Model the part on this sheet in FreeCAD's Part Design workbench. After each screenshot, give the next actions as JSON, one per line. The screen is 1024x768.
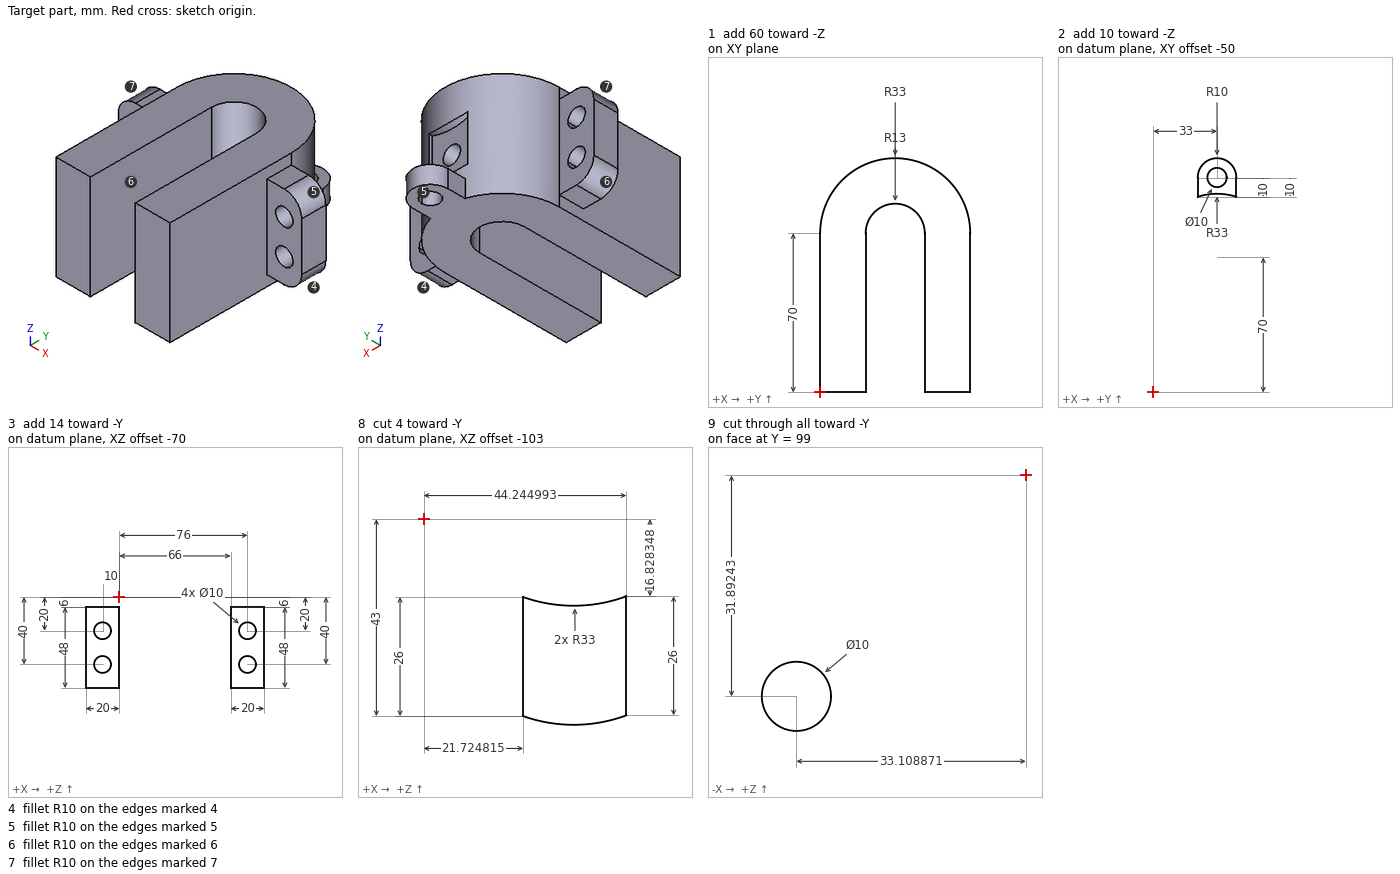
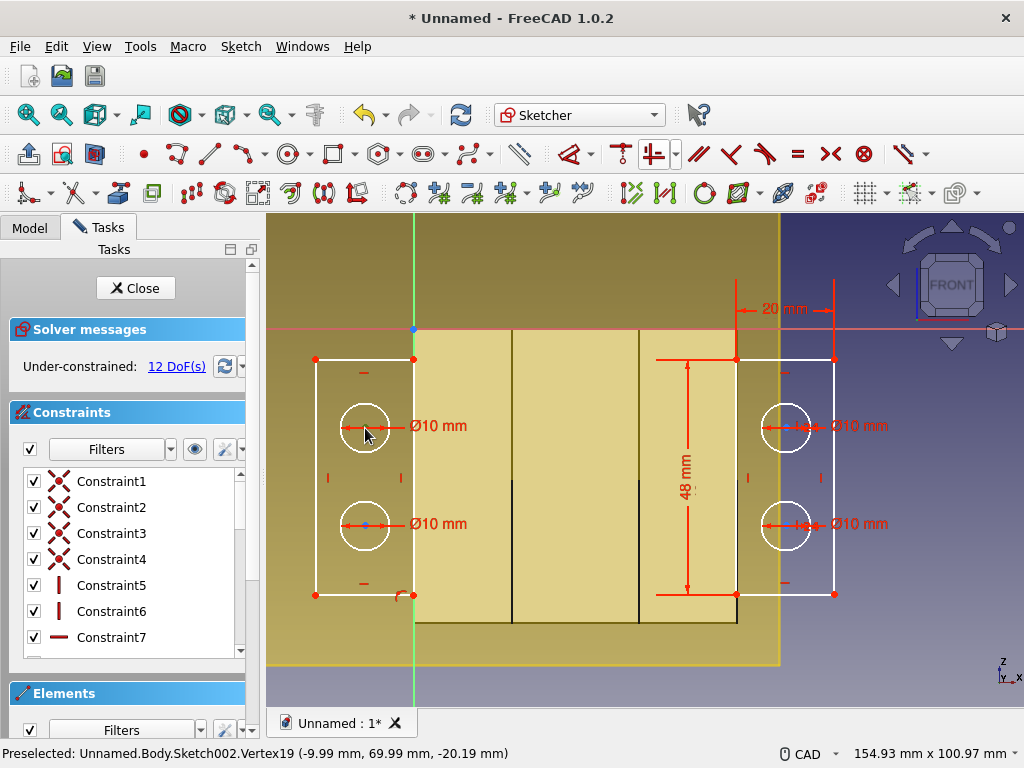
{"action": "left_click", "coordinate": [365, 526]}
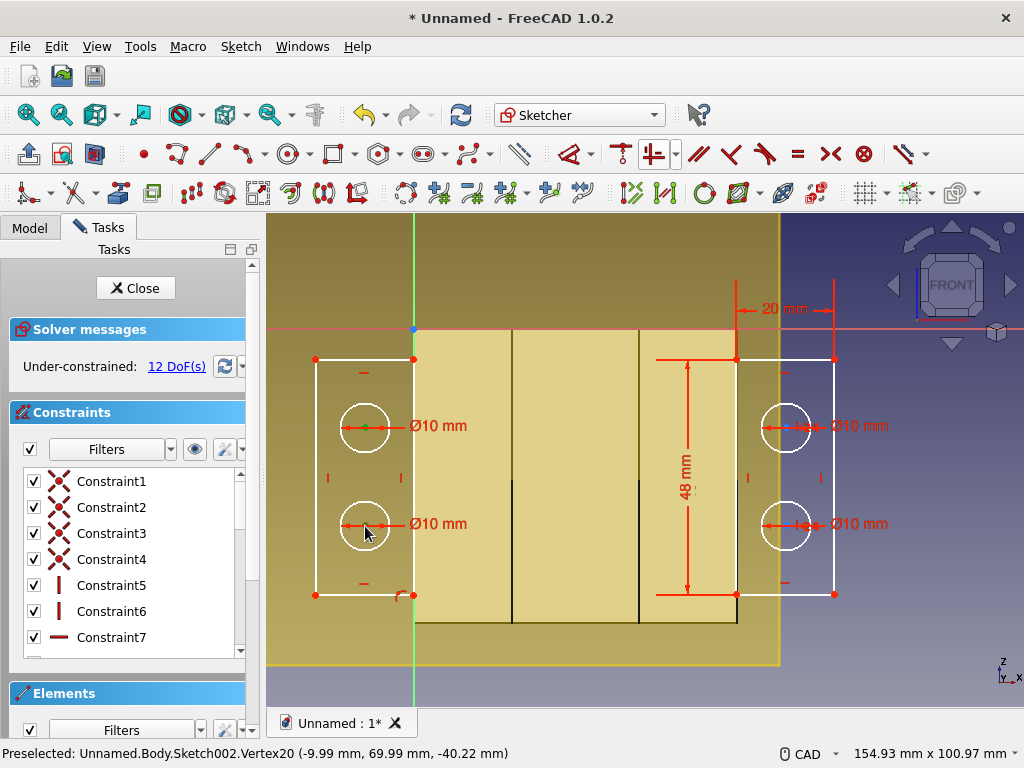
{"action": "key", "text": "v"}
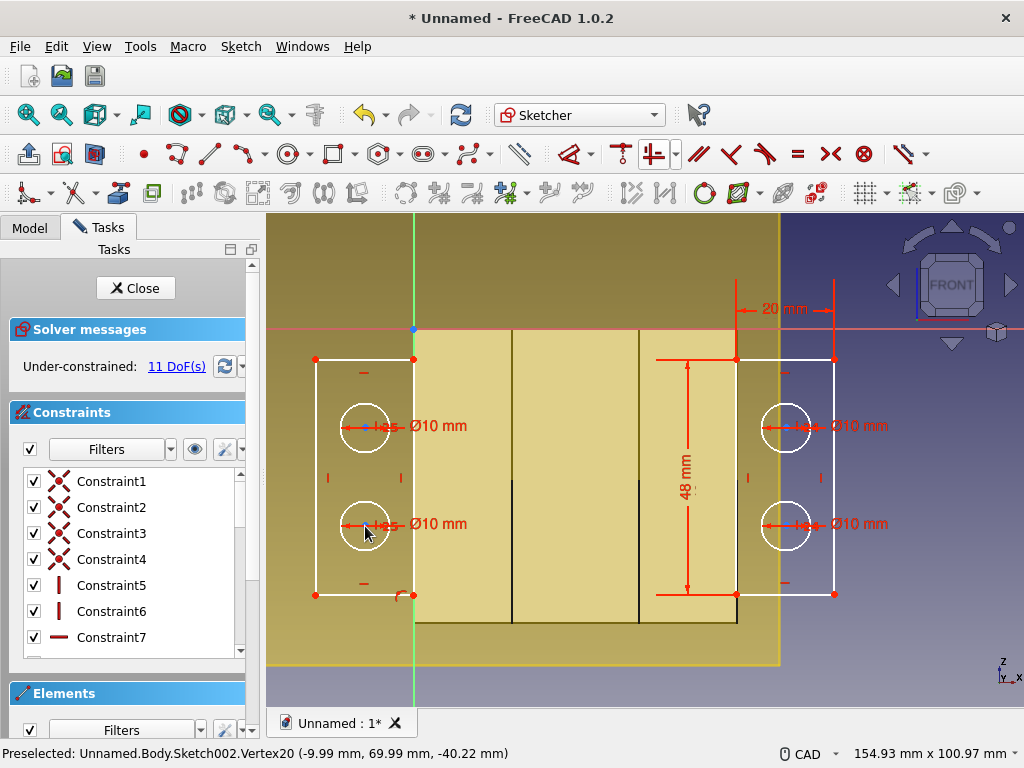
{"action": "left_click", "coordinate": [568, 154]}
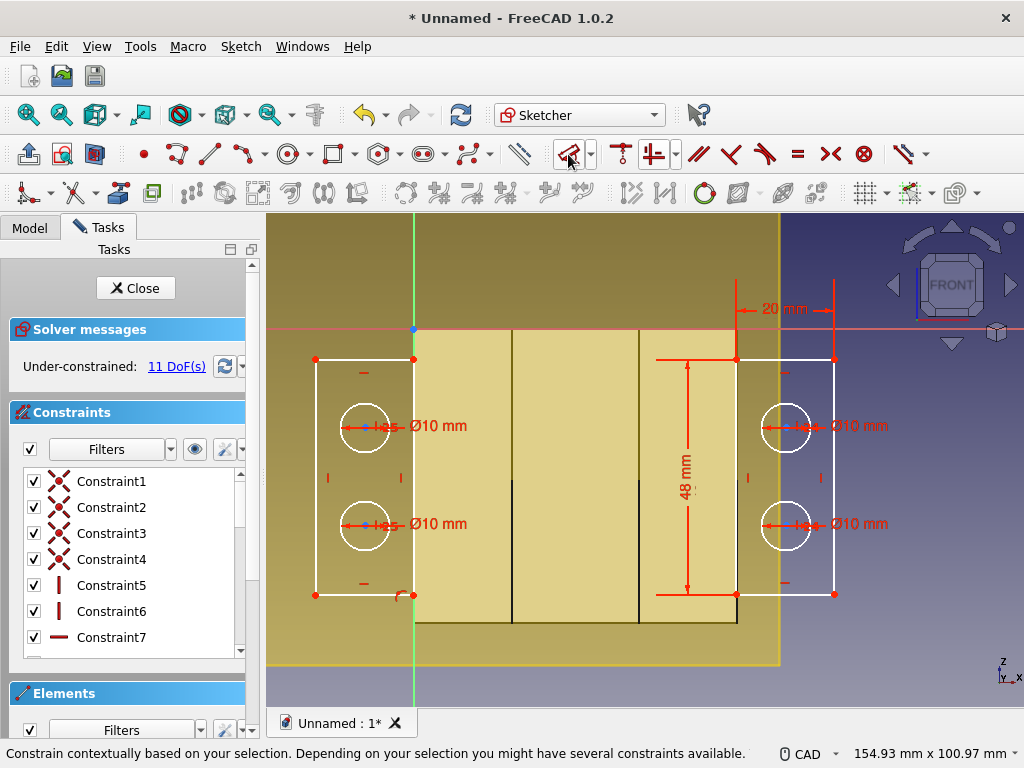
{"action": "left_click", "coordinate": [316, 430]}
{"action": "left_click", "coordinate": [350, 478]}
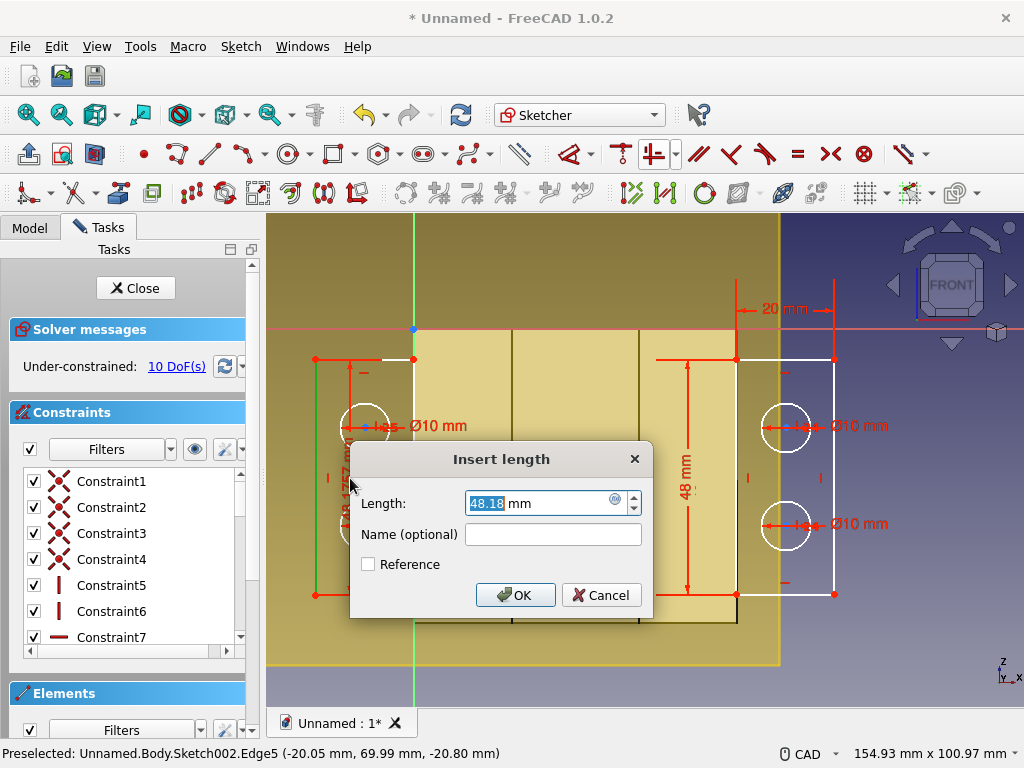
{"action": "type", "text": "48"}
{"action": "key", "text": "Return"}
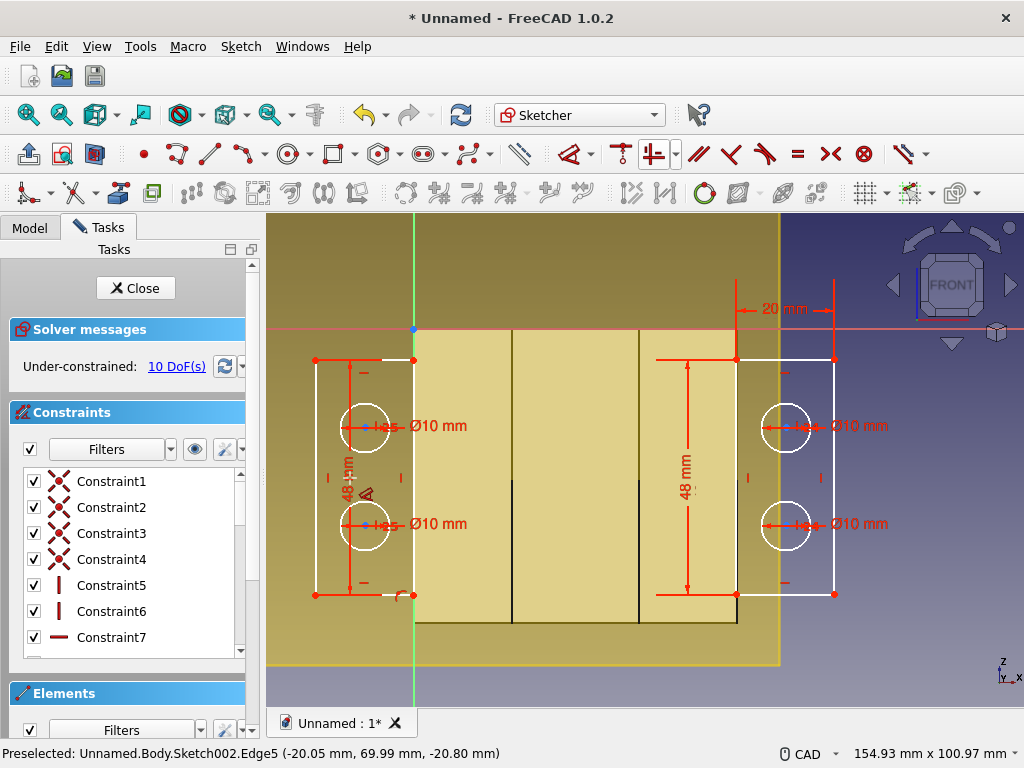
{"action": "left_click", "coordinate": [345, 595]}
{"action": "left_click", "coordinate": [365, 629]}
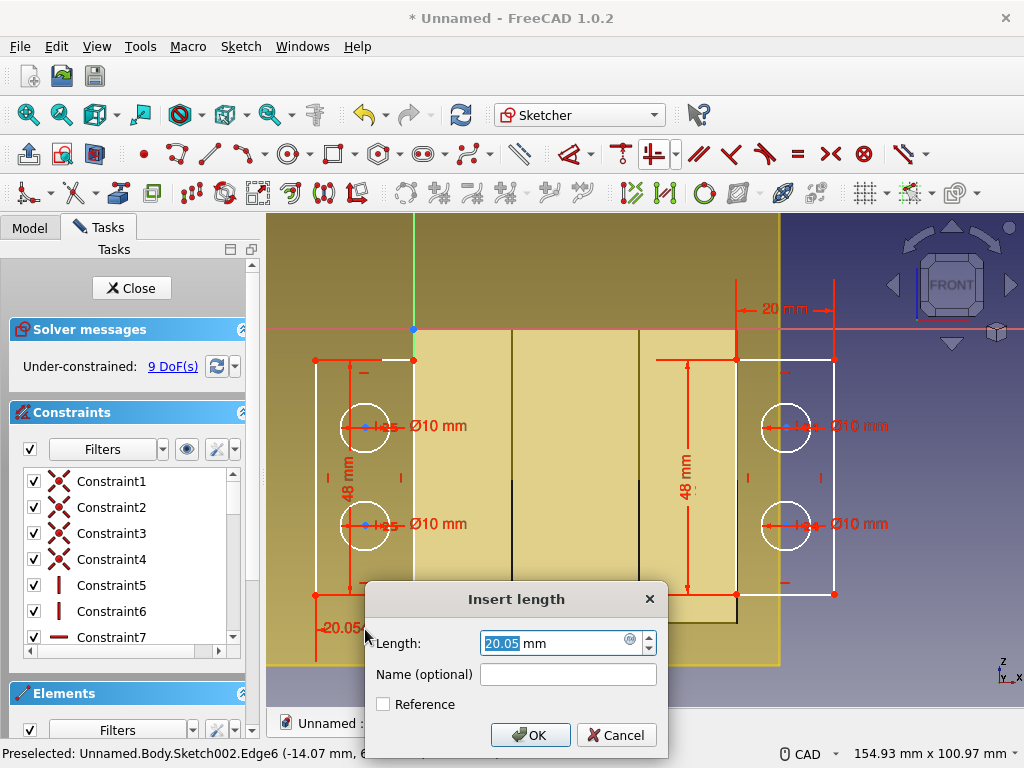
{"action": "type", "text": "20"}
{"action": "key", "text": "Return"}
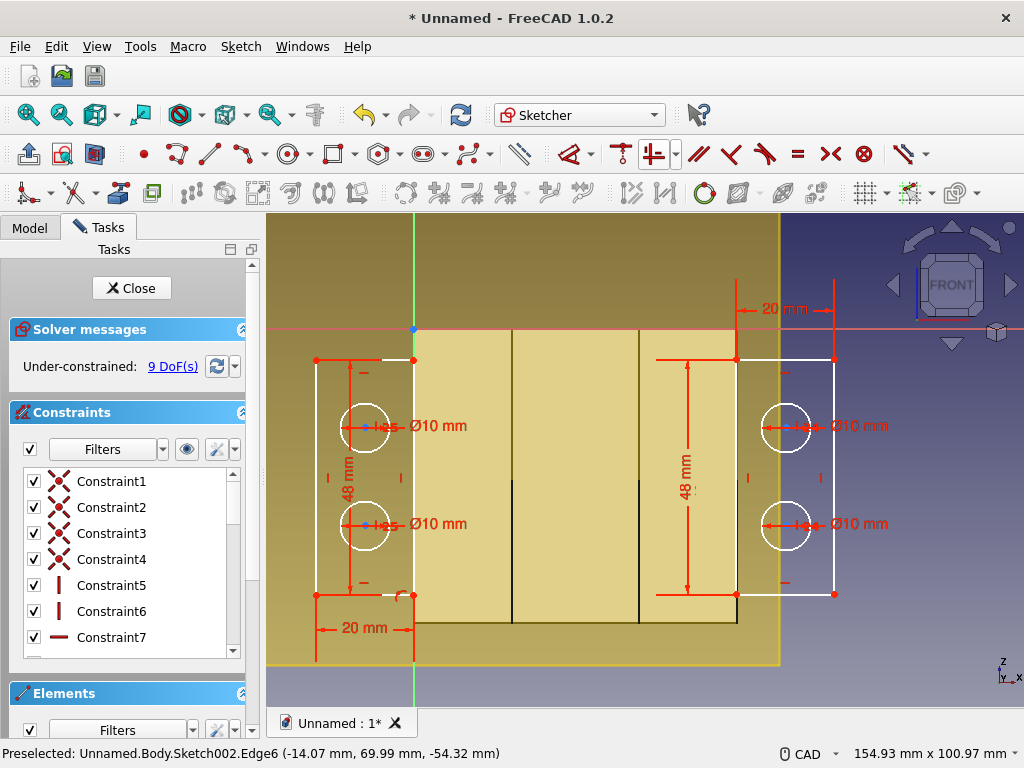
{"action": "scroll", "coordinate": [736, 360], "scroll_direction": "up", "scroll_amount": 2}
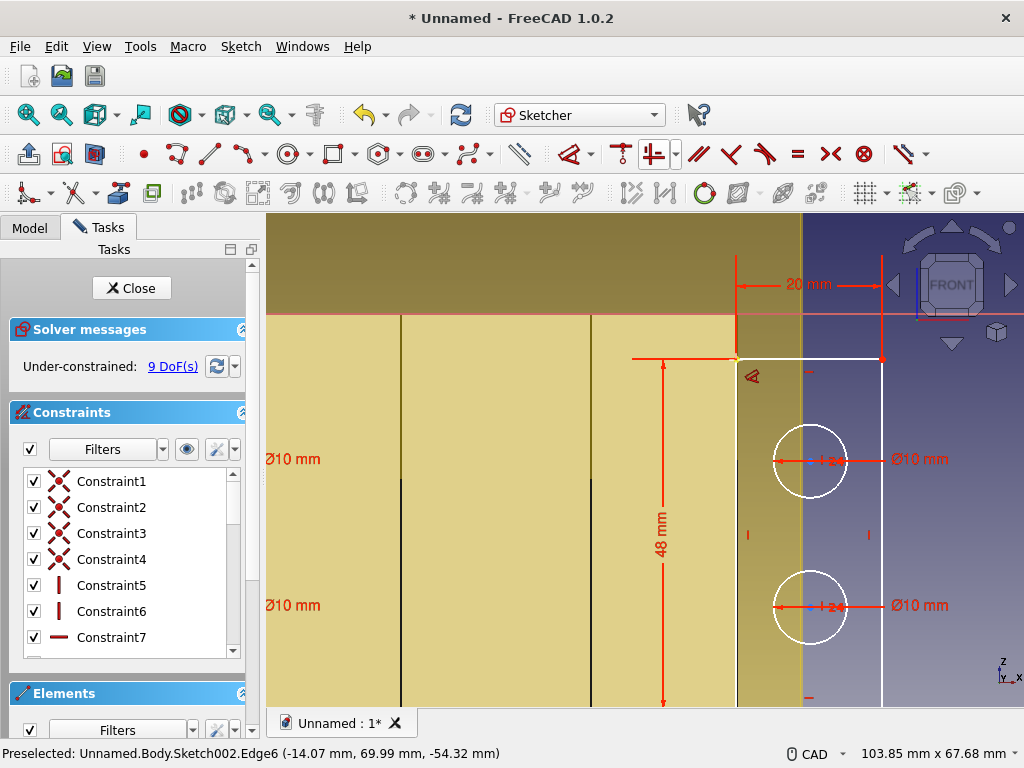
{"action": "left_click", "coordinate": [736, 359]}
{"action": "left_click", "coordinate": [770, 337]}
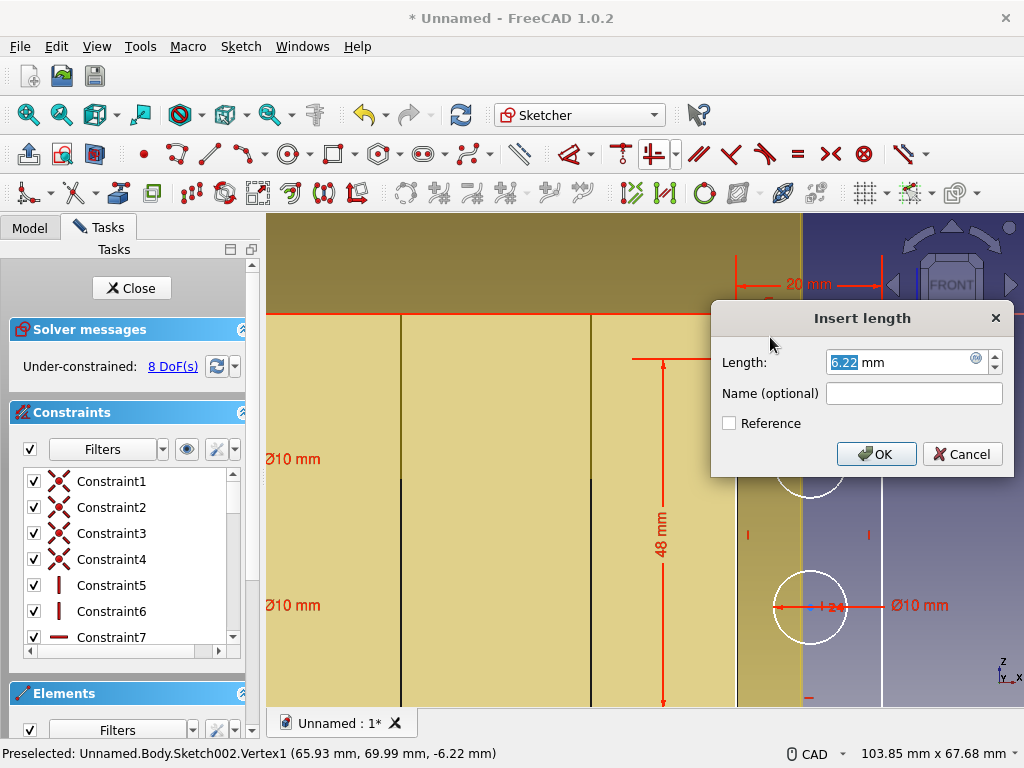
{"action": "type", "text": "6"}
{"action": "key", "text": "Return"}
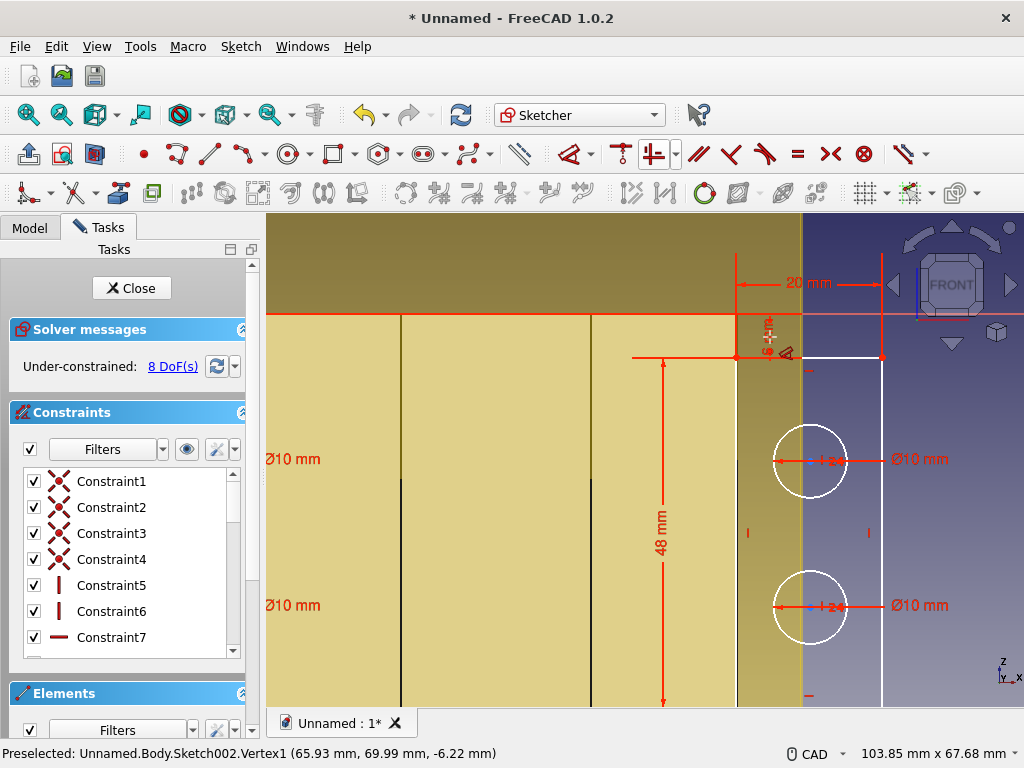
{"action": "scroll", "coordinate": [674, 398], "scroll_direction": "down", "scroll_amount": 3}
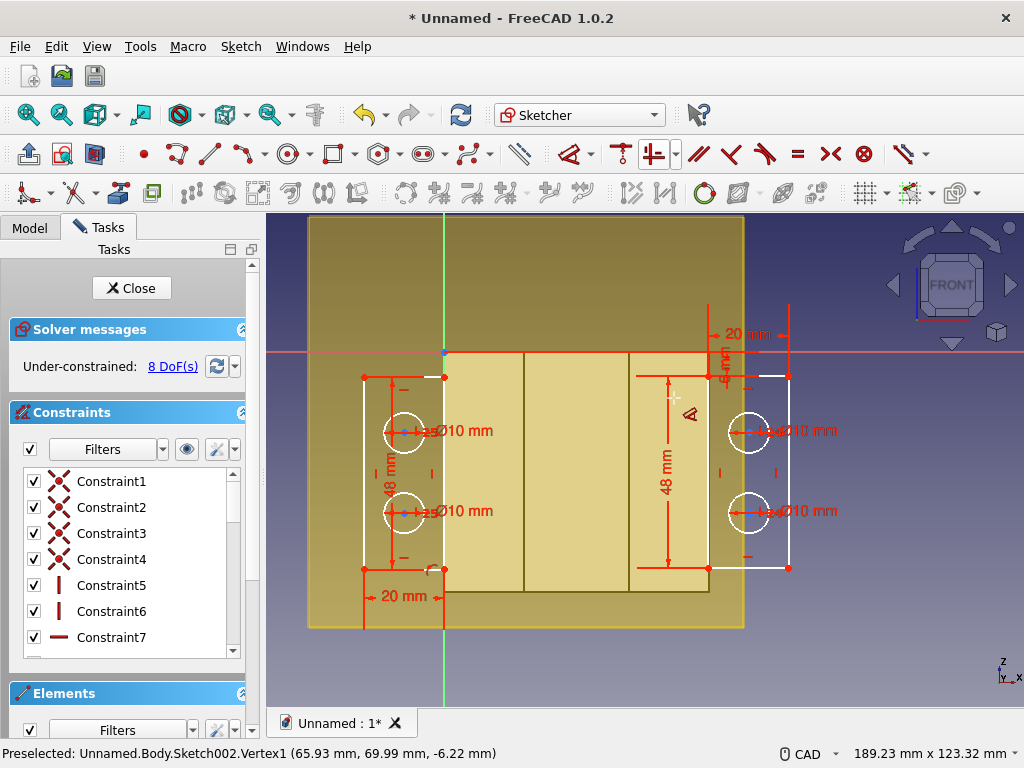
{"action": "scroll", "coordinate": [364, 377], "scroll_direction": "up", "scroll_amount": 3}